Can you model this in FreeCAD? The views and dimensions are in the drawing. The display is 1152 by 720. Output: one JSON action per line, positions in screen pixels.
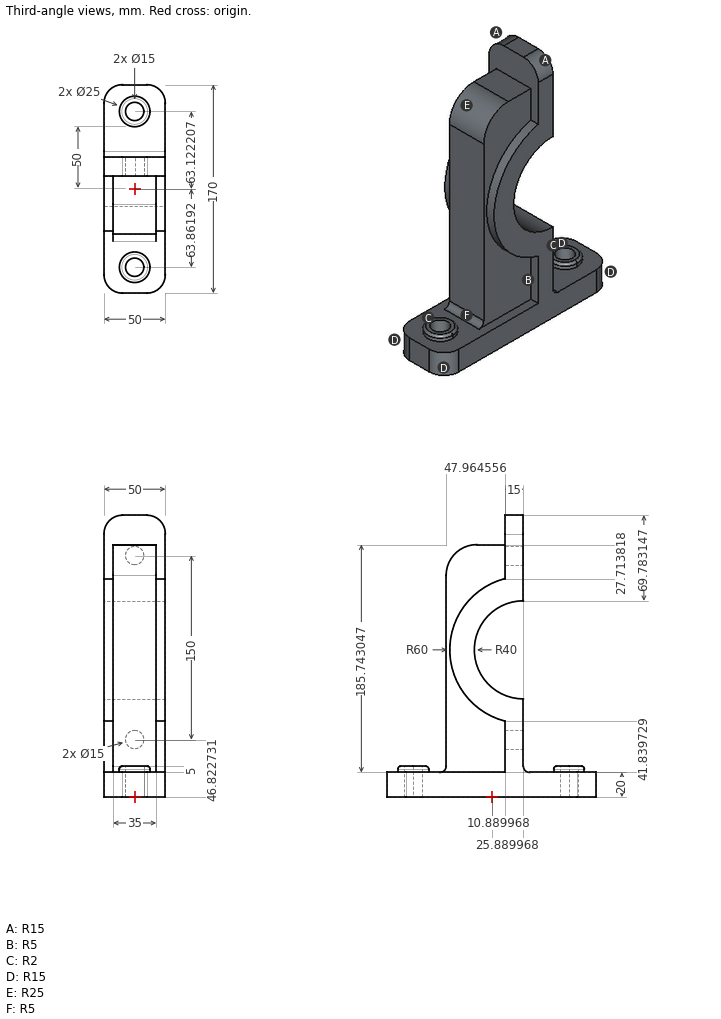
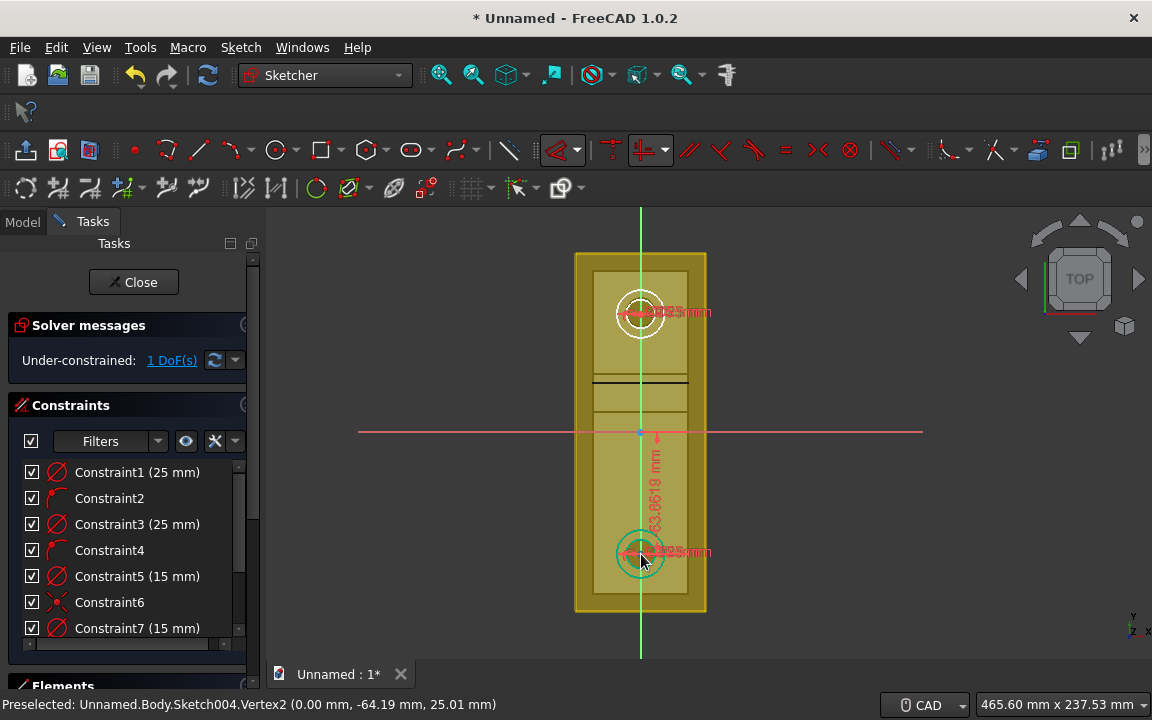
{"action": "left_click", "coordinate": [641, 314]}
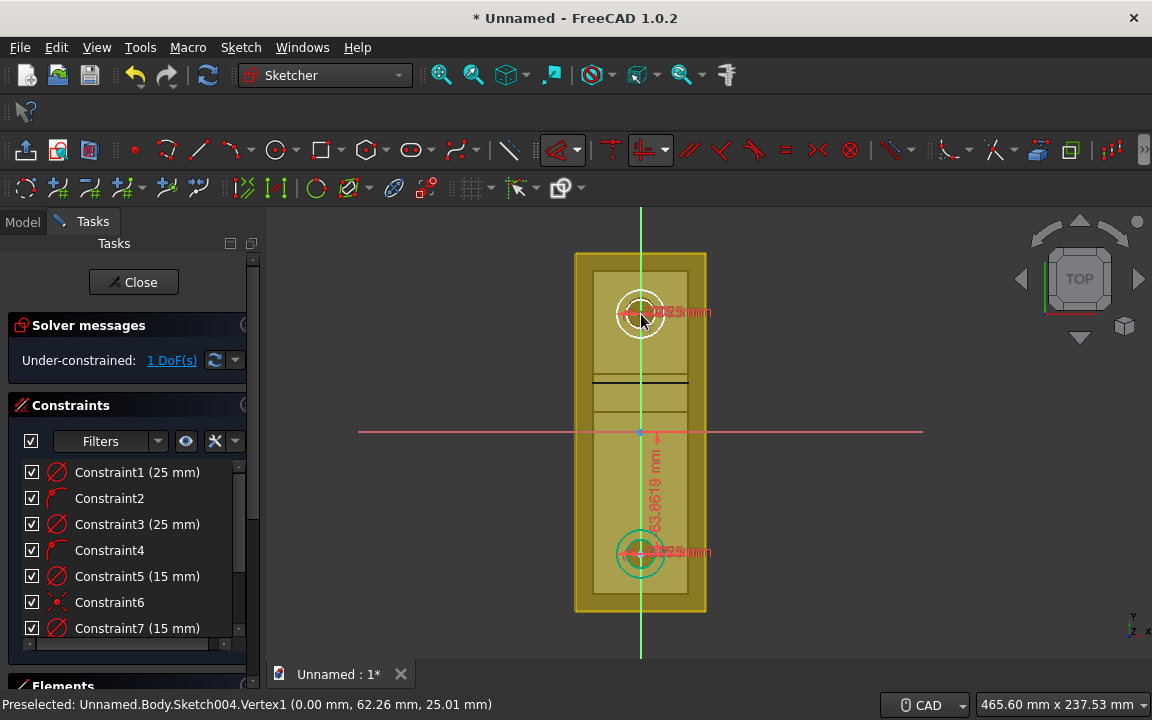
{"action": "key", "text": "i"}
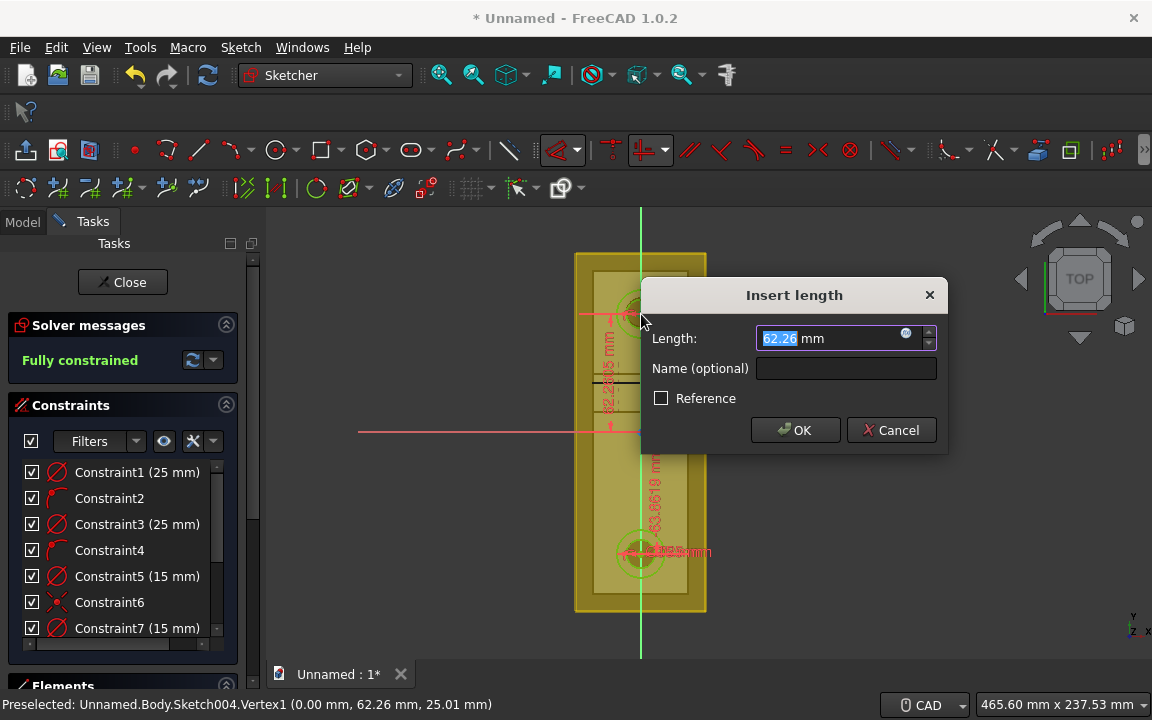
{"action": "type", "text": "63.122207"}
{"action": "key", "text": "Return"}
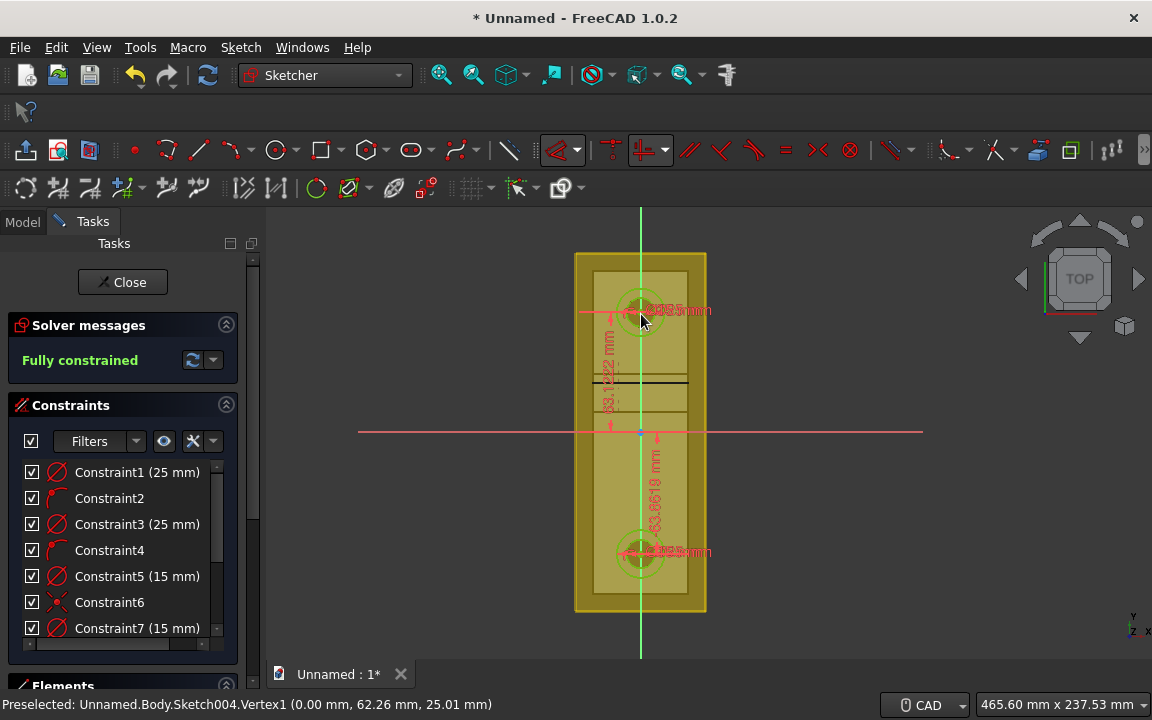
{"action": "left_click", "coordinate": [123, 282]}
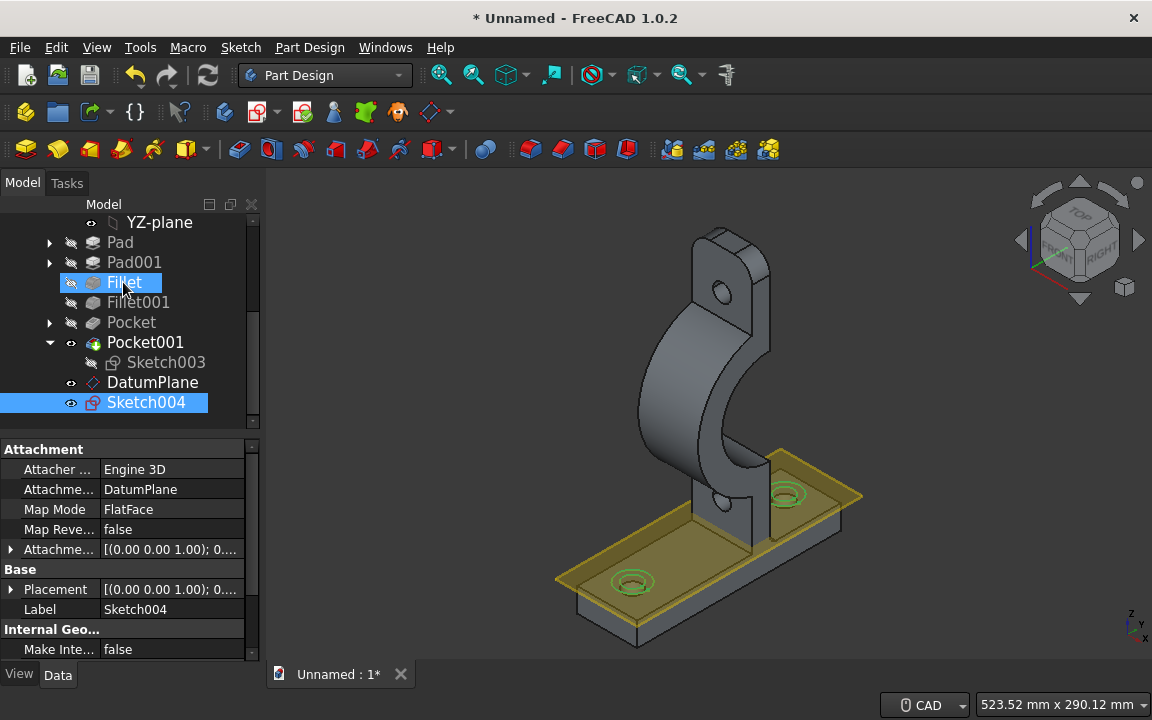
{"action": "left_click", "coordinate": [26, 150]}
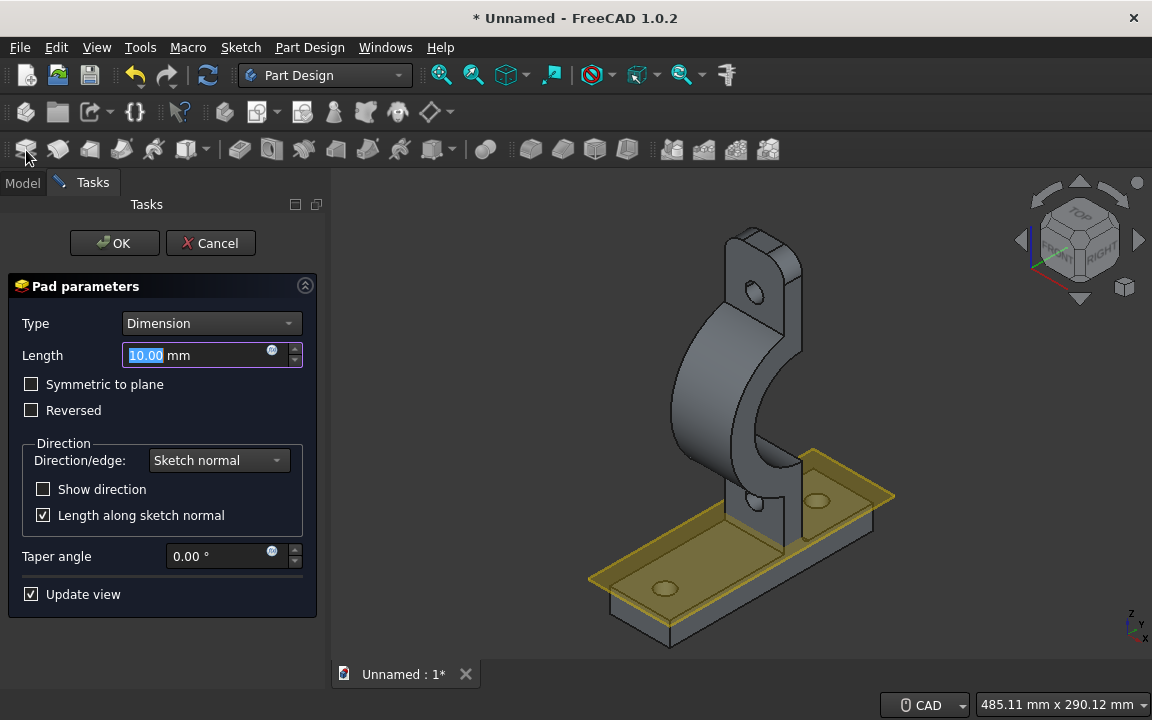
{"action": "type", "text": "5"}
{"action": "key", "text": "Tab"}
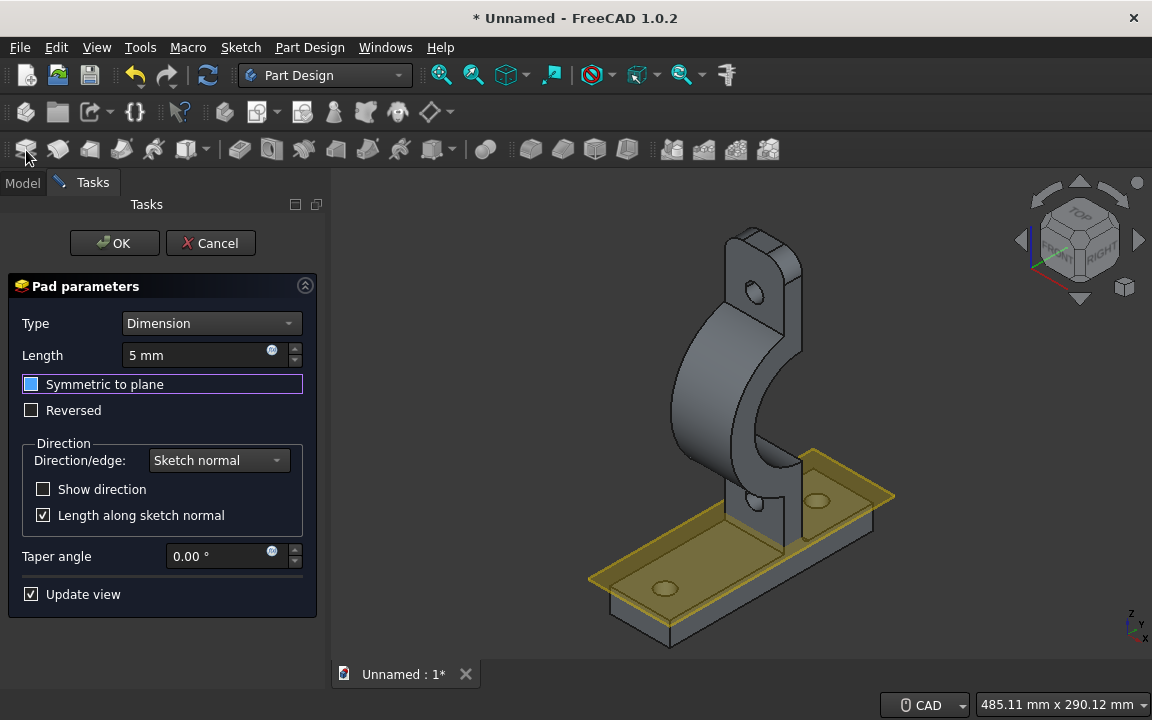
{"action": "left_click", "coordinate": [30, 410]}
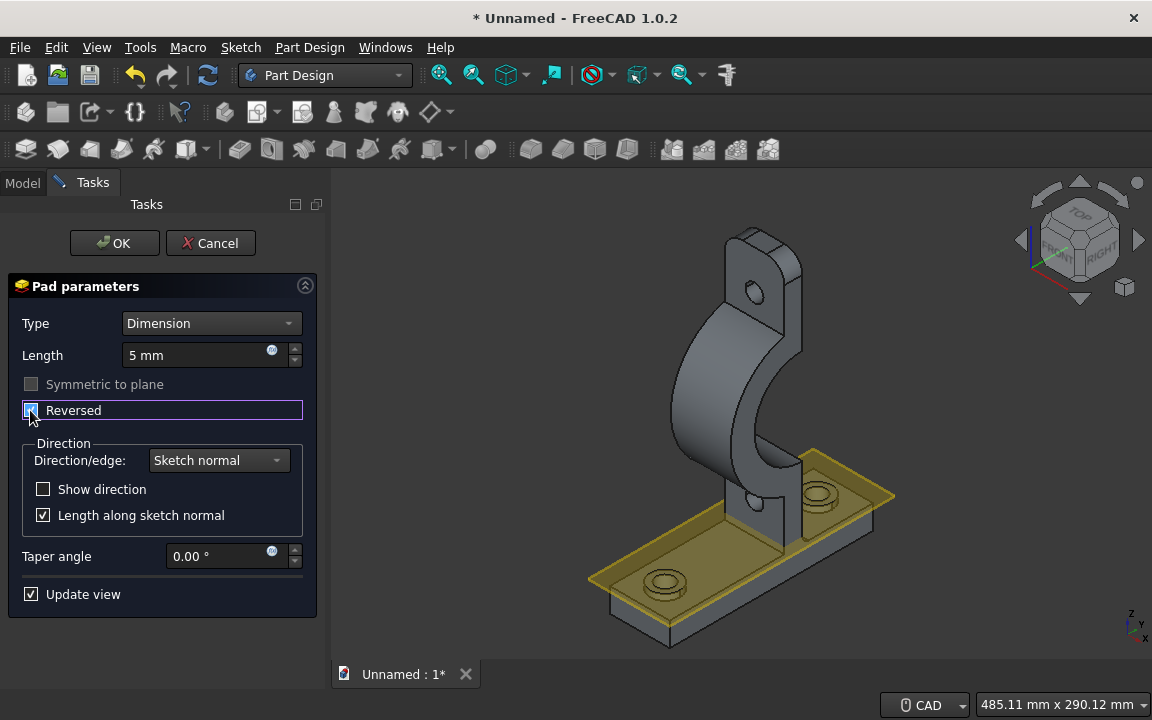
{"action": "left_click", "coordinate": [115, 243]}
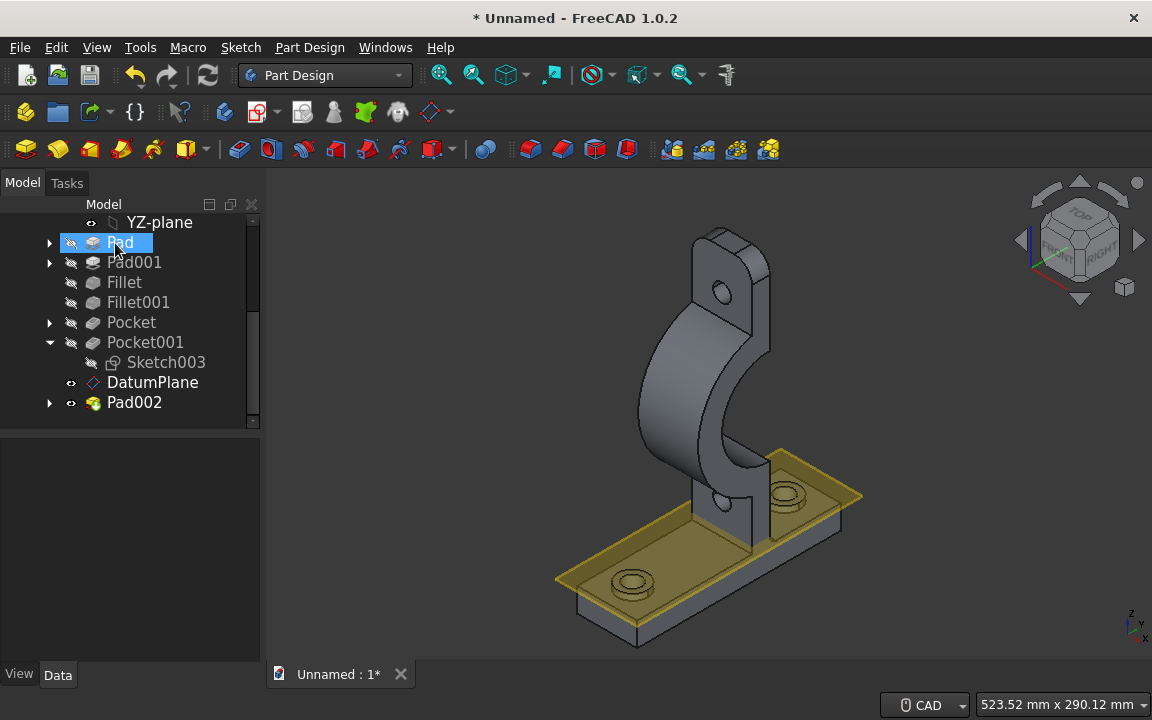
{"action": "left_click", "coordinate": [116, 383]}
{"action": "key", "text": "space"}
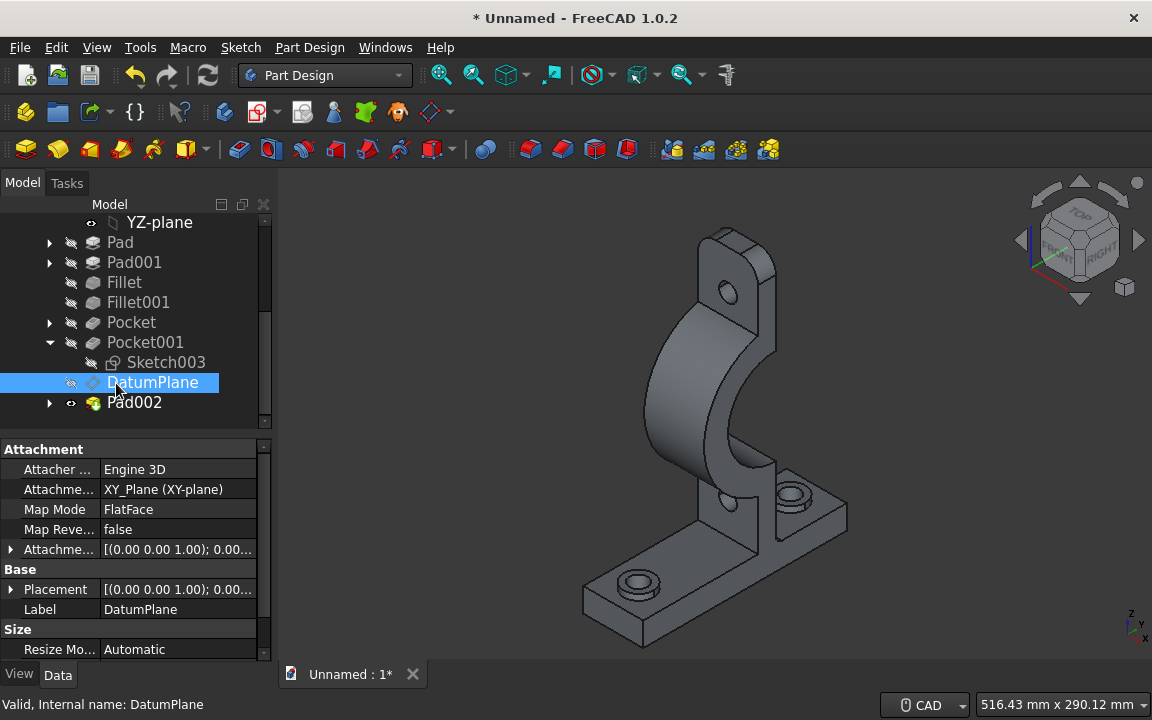
{"action": "left_click", "coordinate": [809, 488]}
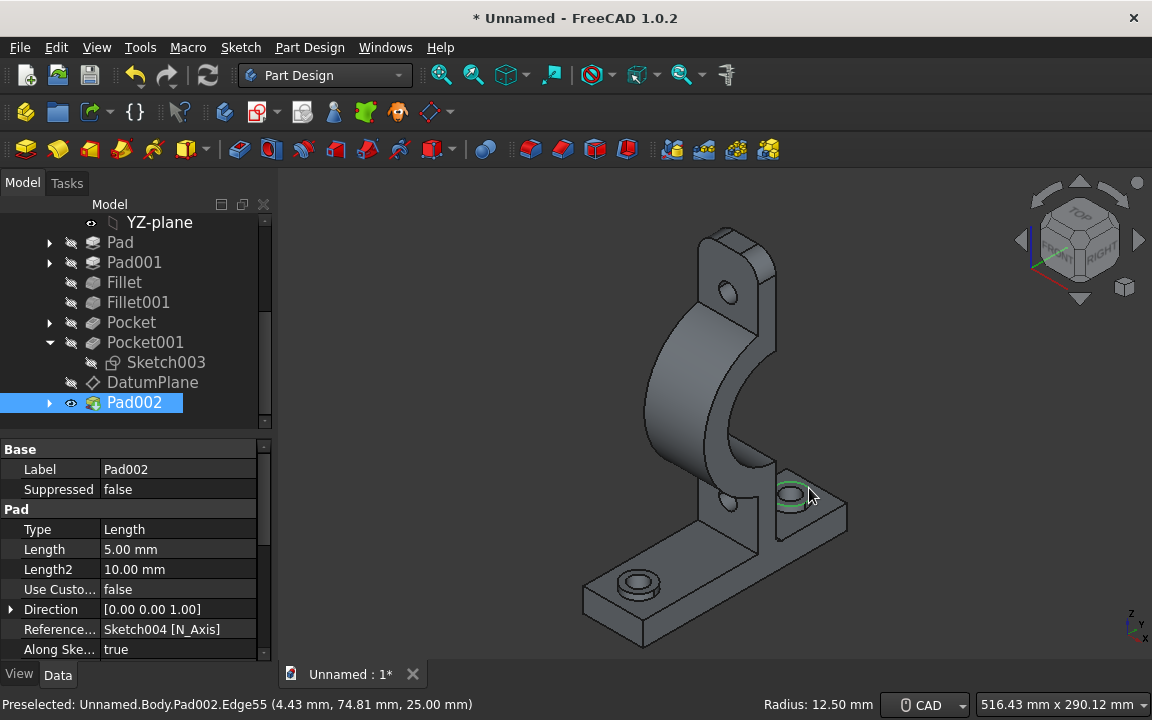
{"action": "left_click", "coordinate": [618, 579], "text": "ctrl"}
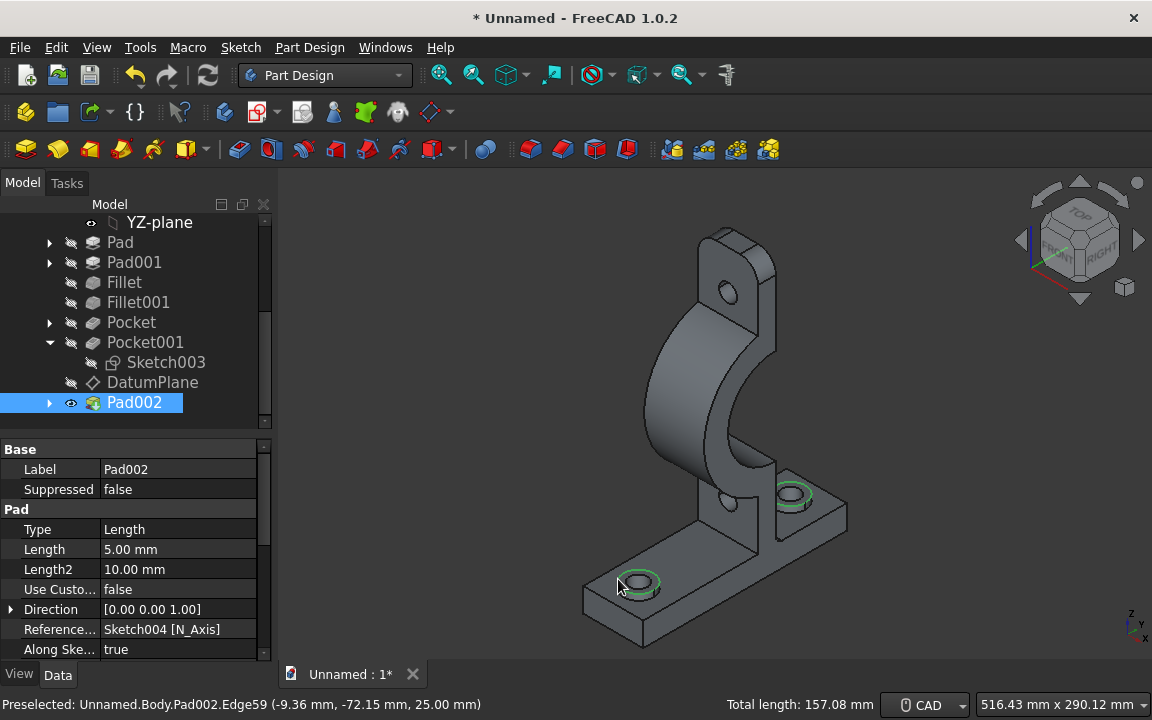
{"action": "left_click", "coordinate": [532, 150]}